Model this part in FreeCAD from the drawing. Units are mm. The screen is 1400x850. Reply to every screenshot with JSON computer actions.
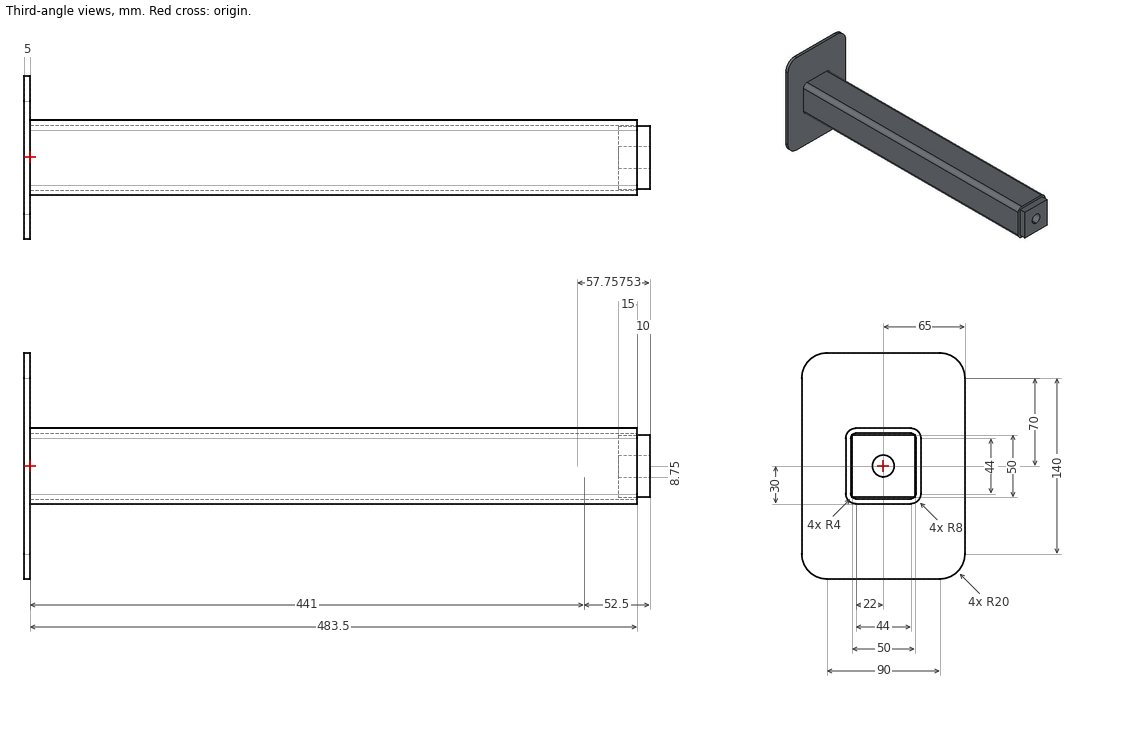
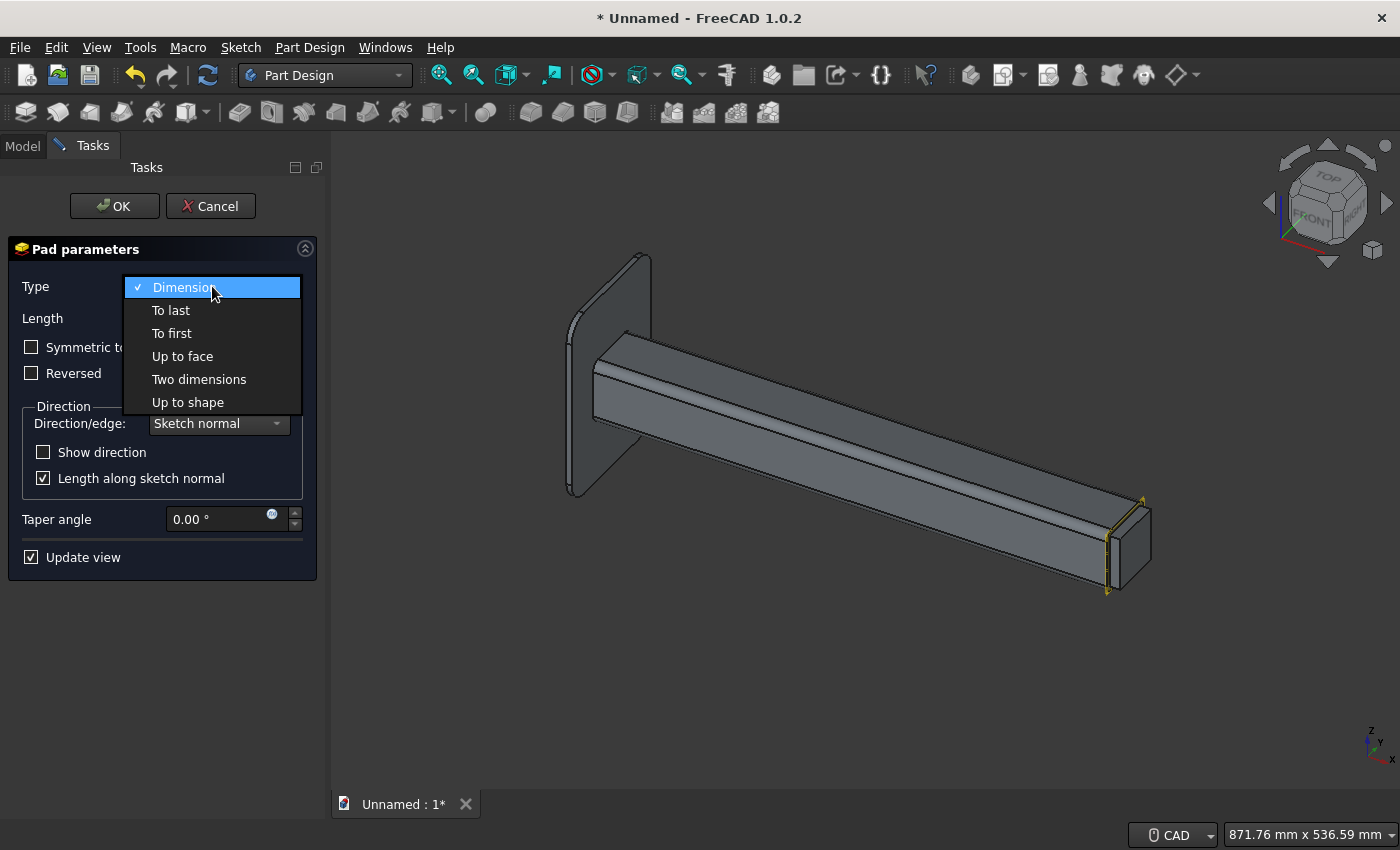
{"action": "left_click", "coordinate": [212, 380]}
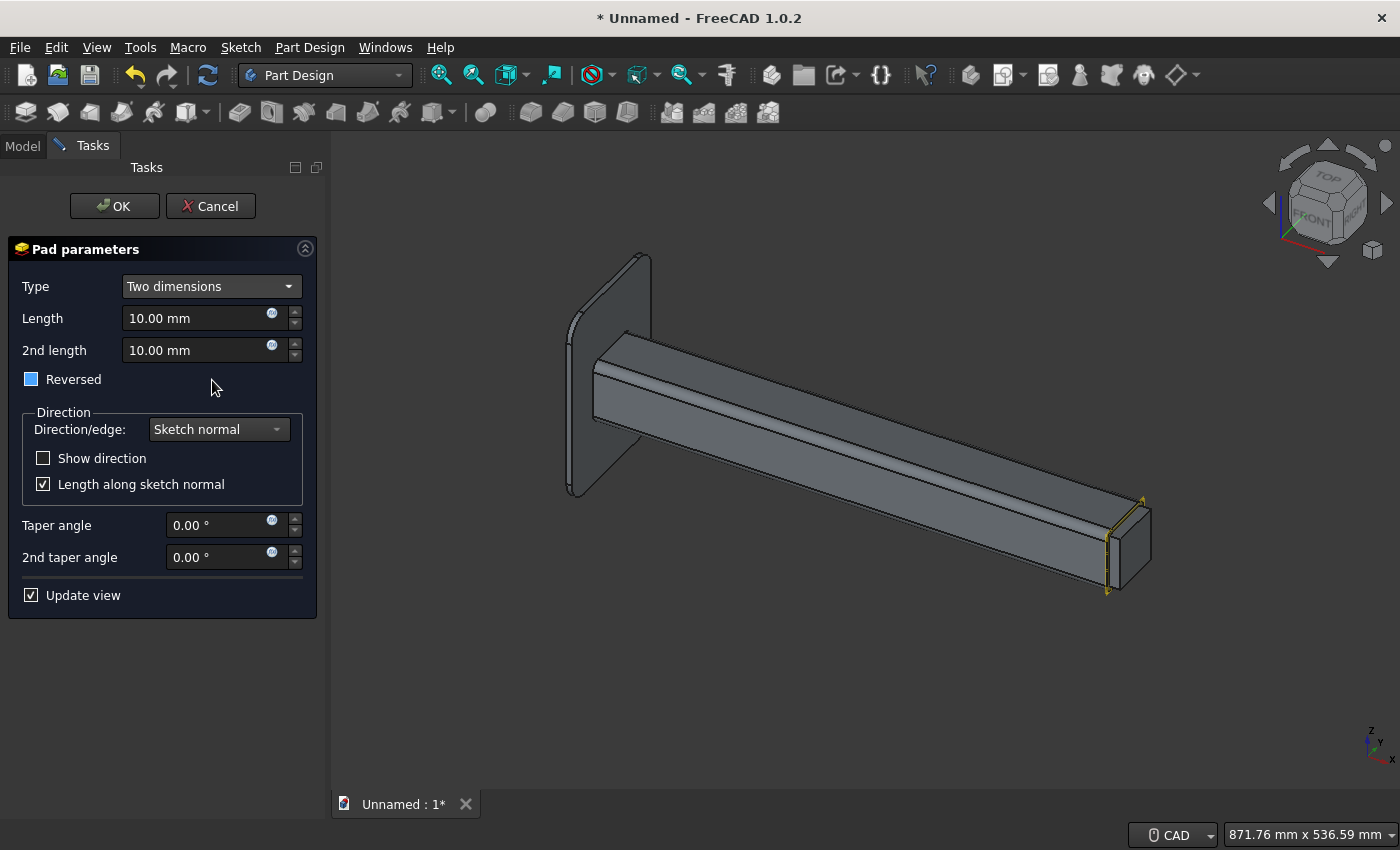
{"action": "triple_click", "coordinate": [204, 318]}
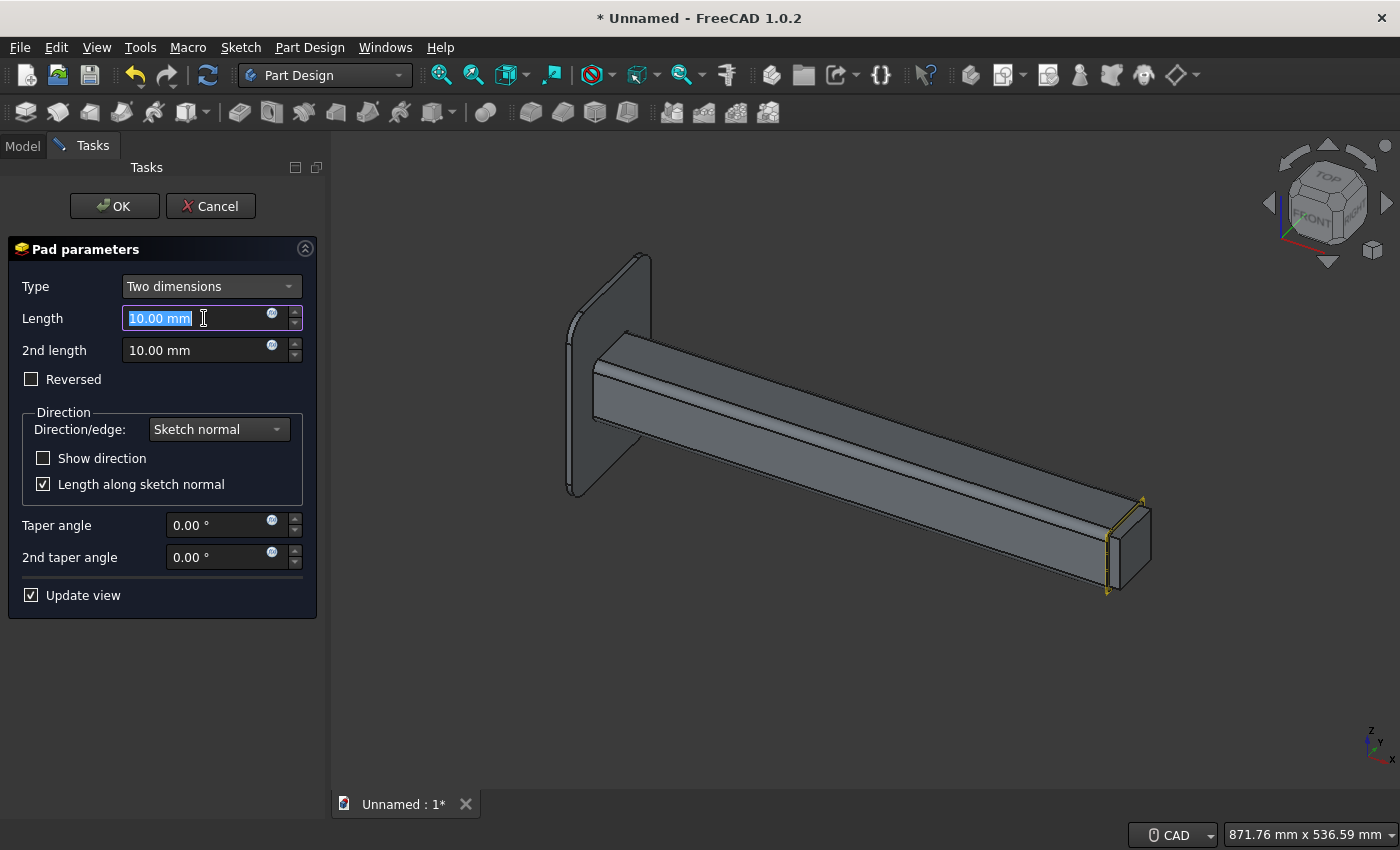
{"action": "type", "text": "10"}
{"action": "key", "text": "Tab"}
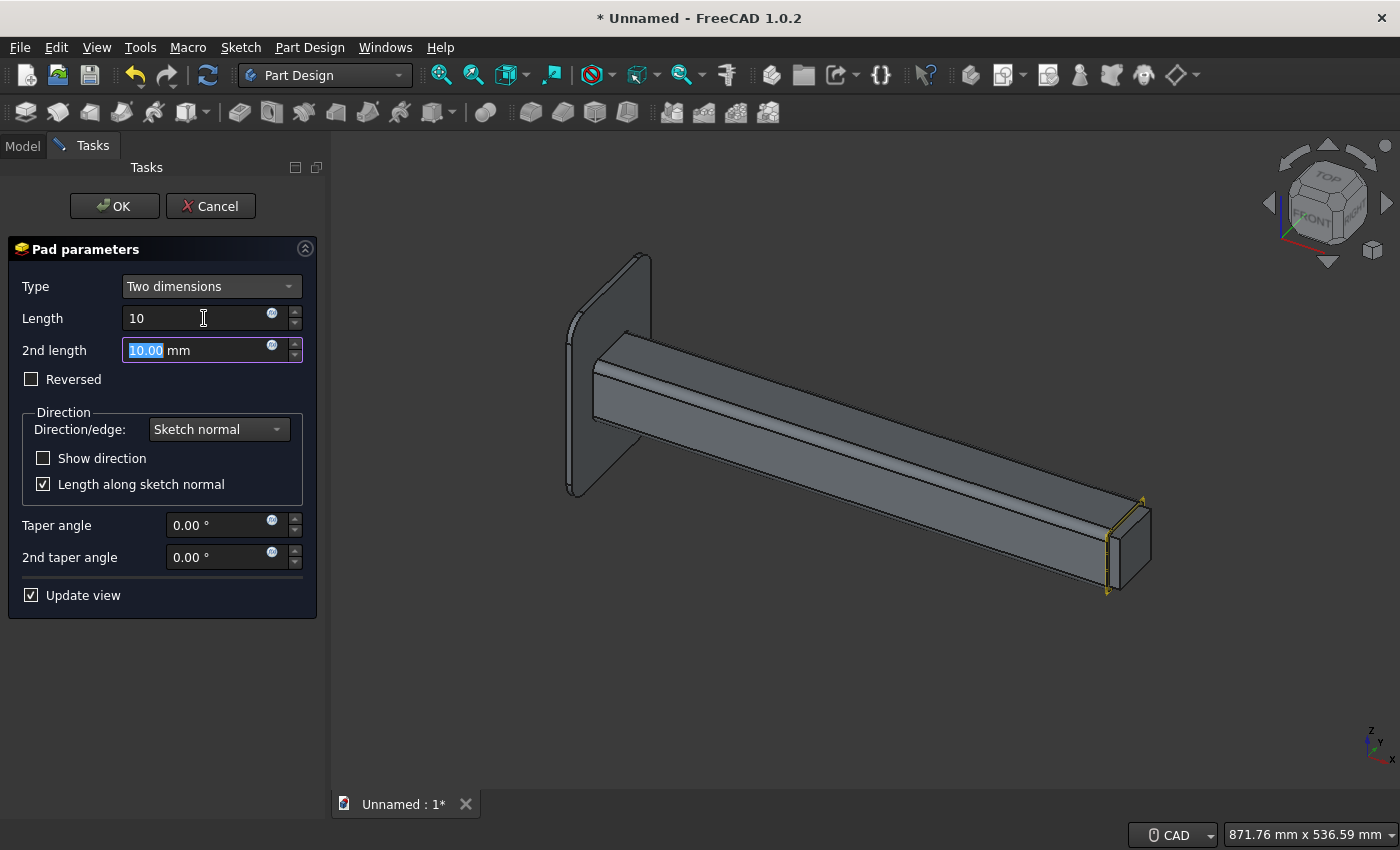
{"action": "type", "text": "15"}
{"action": "key", "text": "Tab"}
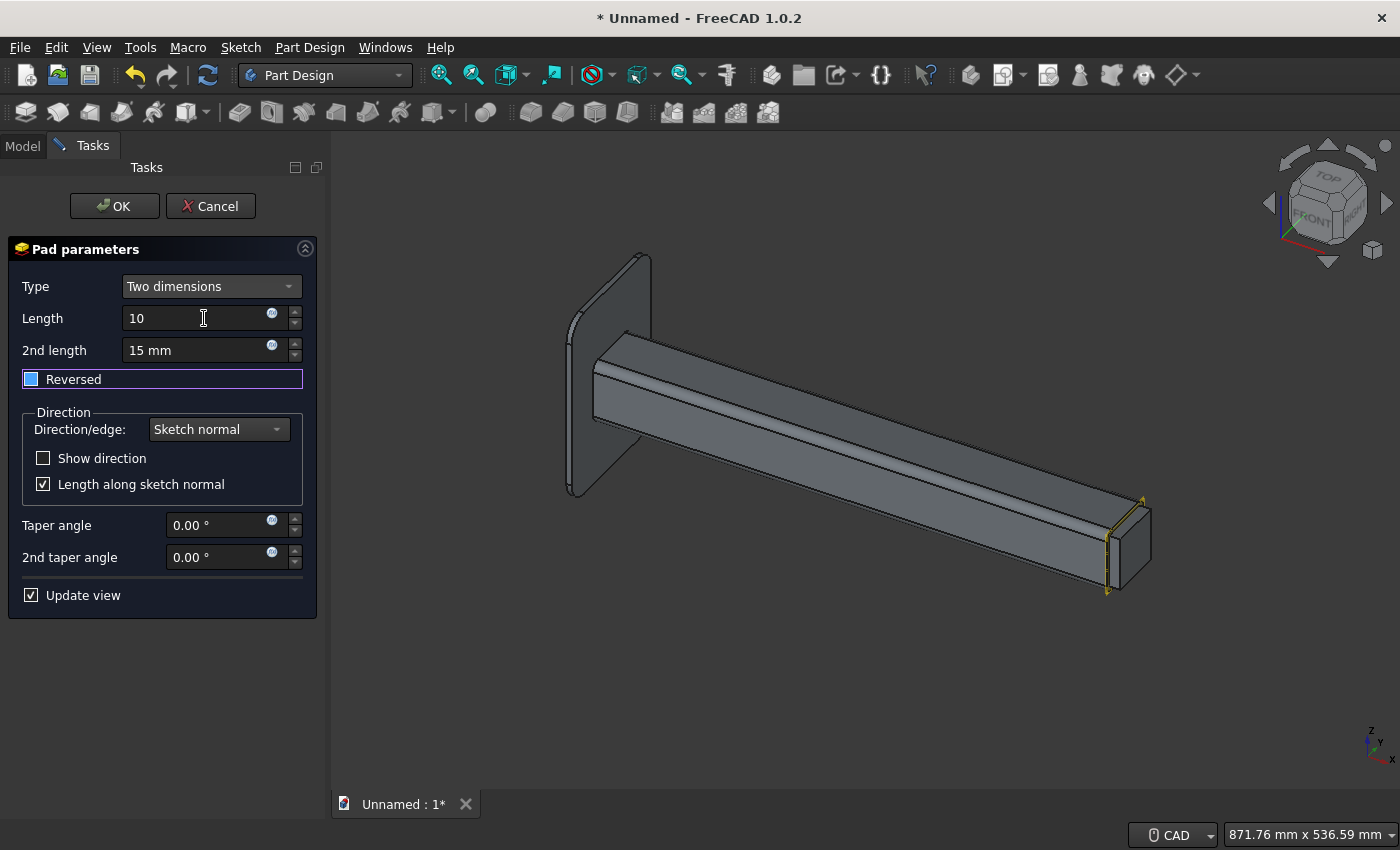
{"action": "left_click", "coordinate": [115, 206]}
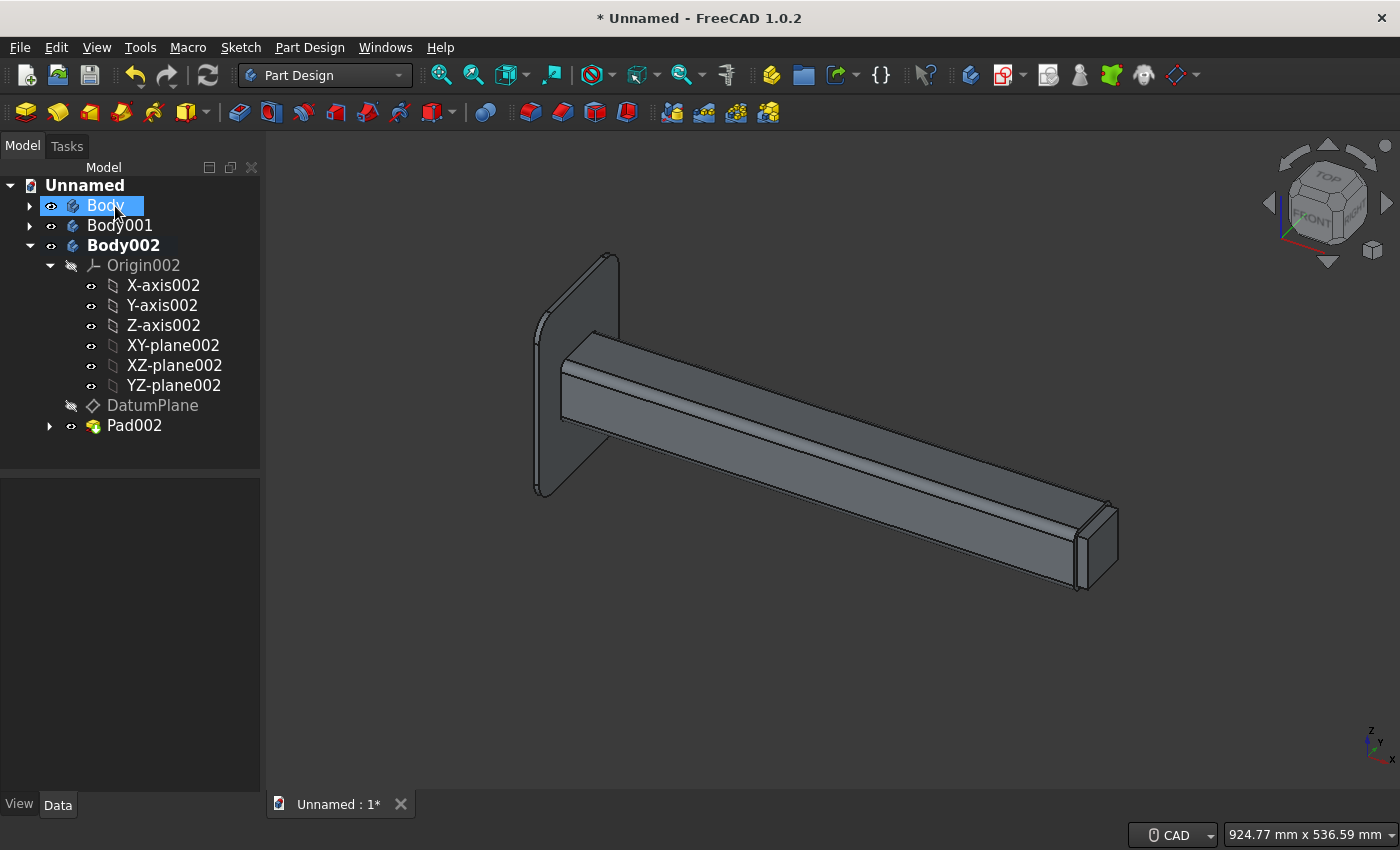
{"action": "left_click", "coordinate": [442, 76]}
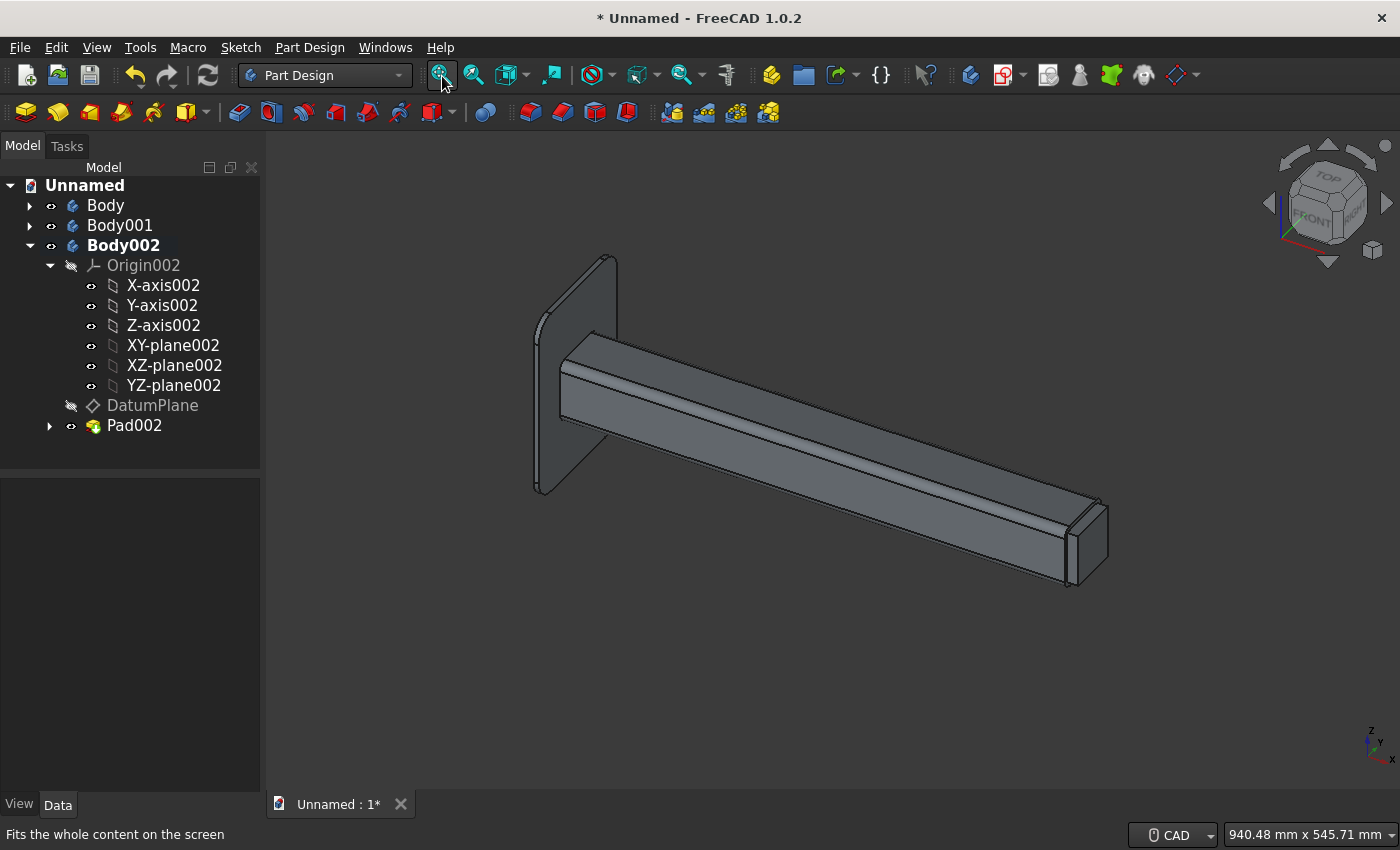
{"action": "left_click", "coordinate": [1004, 76]}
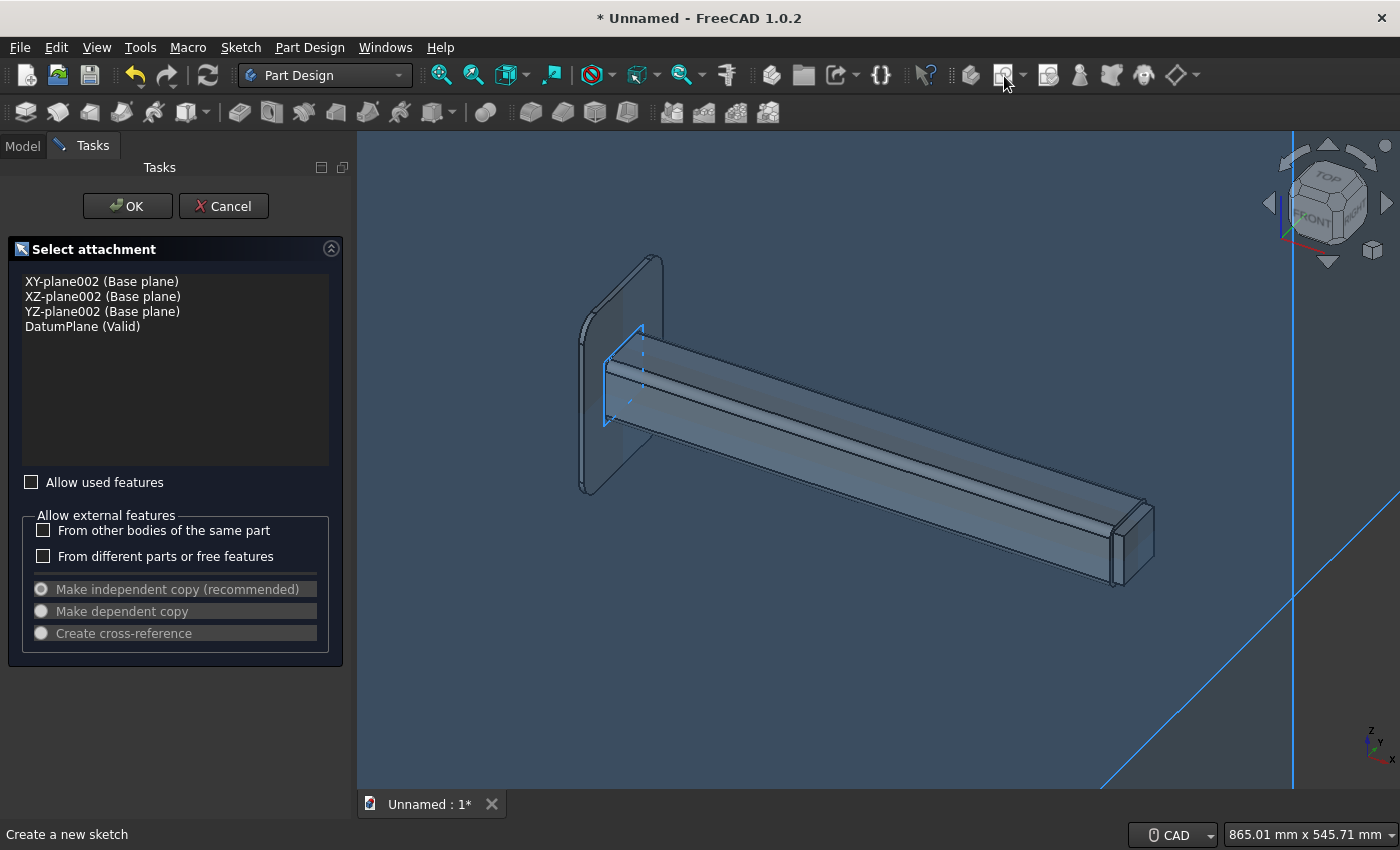
{"action": "left_click", "coordinate": [82, 296]}